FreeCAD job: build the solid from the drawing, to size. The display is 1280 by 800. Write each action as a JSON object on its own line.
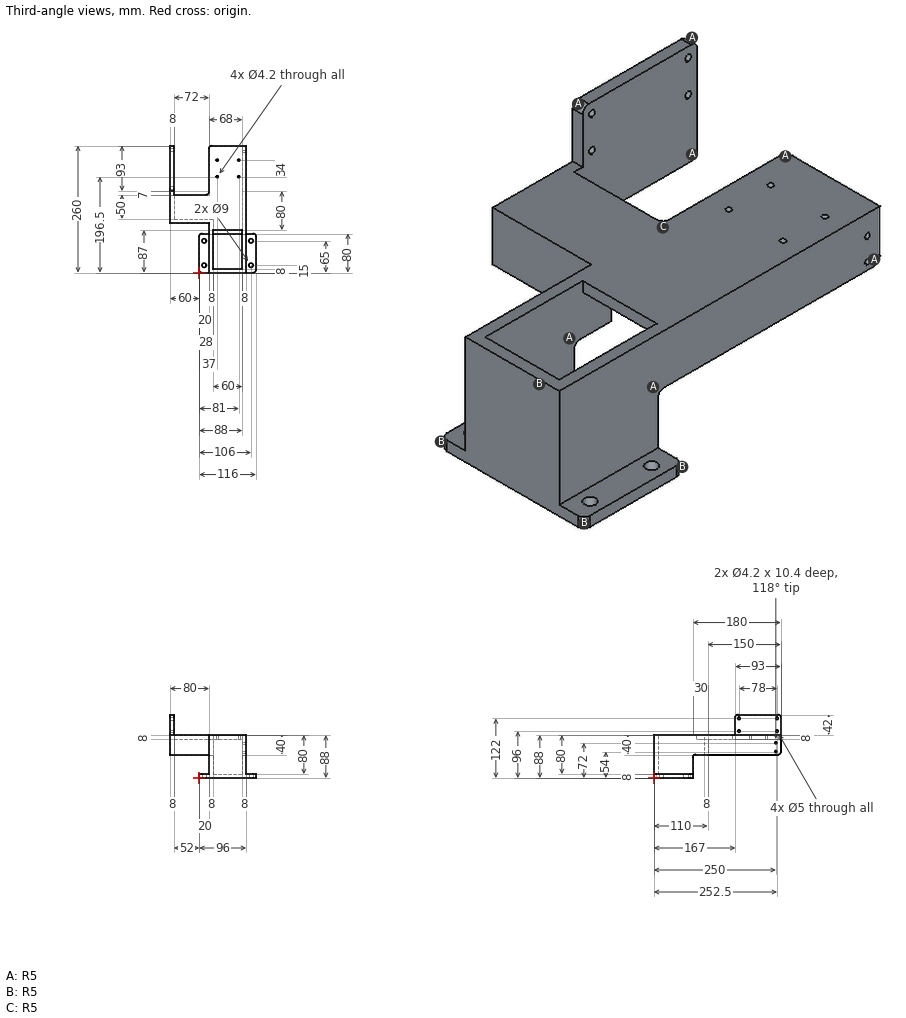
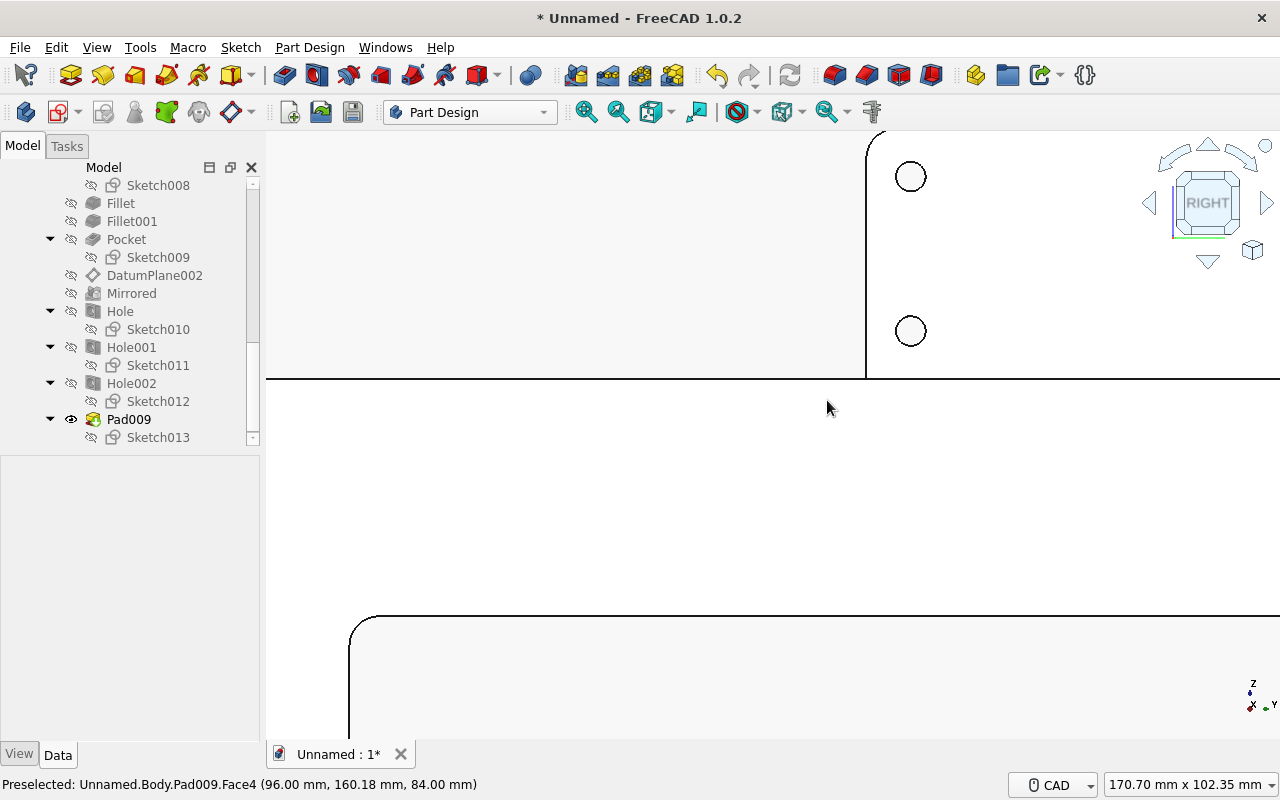
{"action": "left_click", "coordinate": [588, 112]}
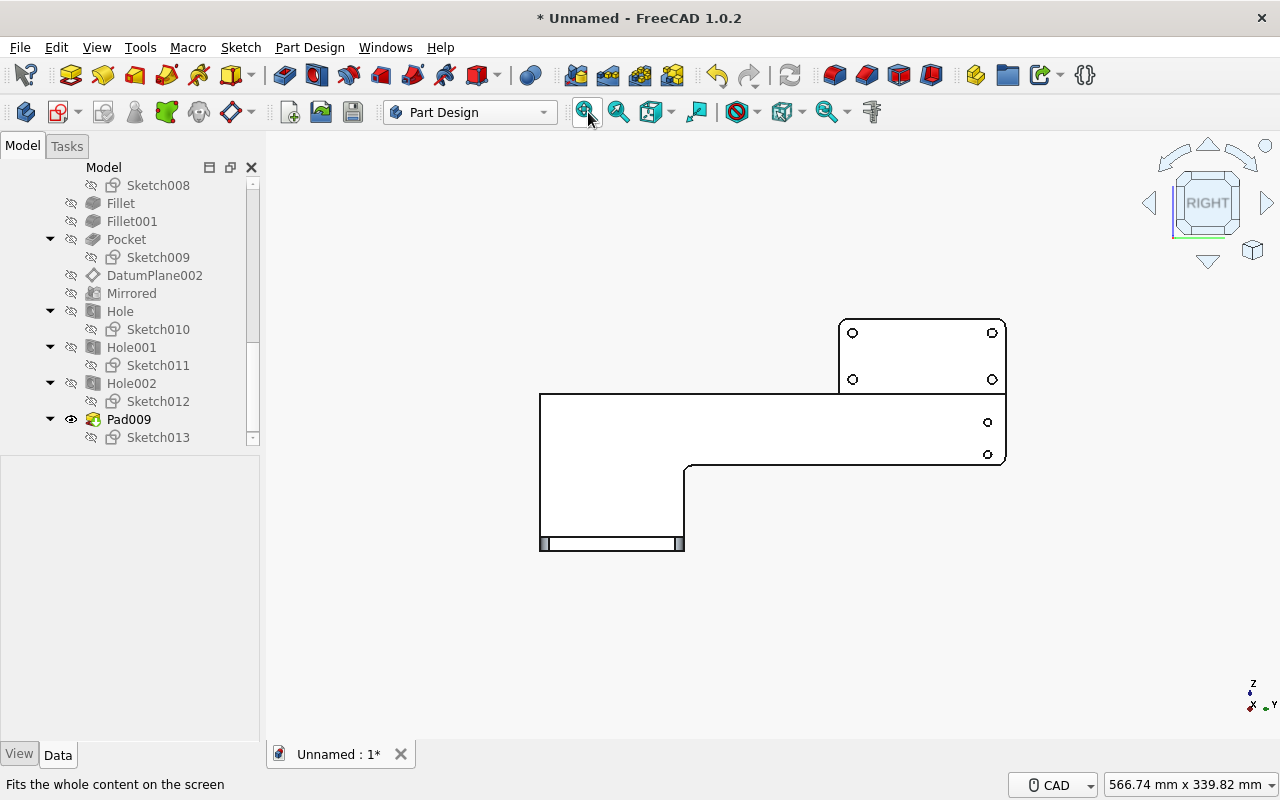
{"action": "key", "text": "5"}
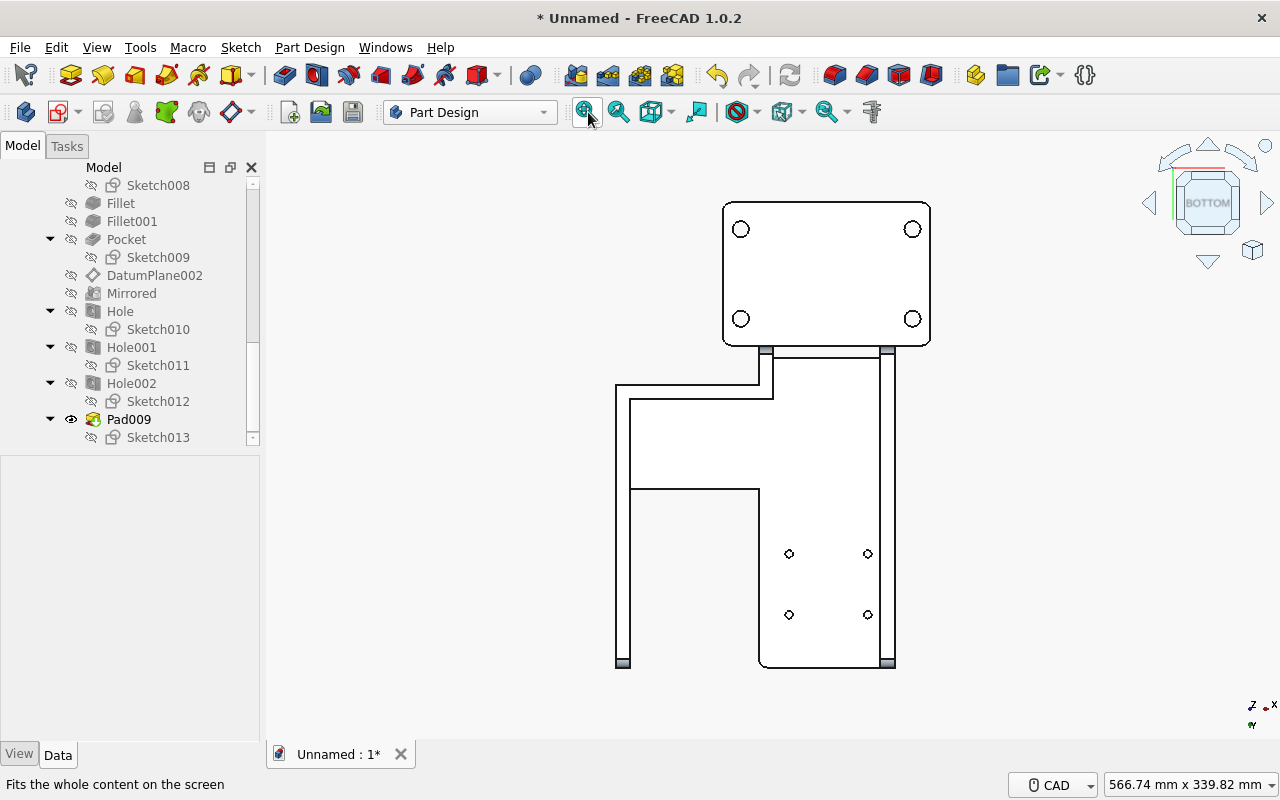
{"action": "scroll", "coordinate": [759, 488], "scroll_direction": "up", "scroll_amount": 6}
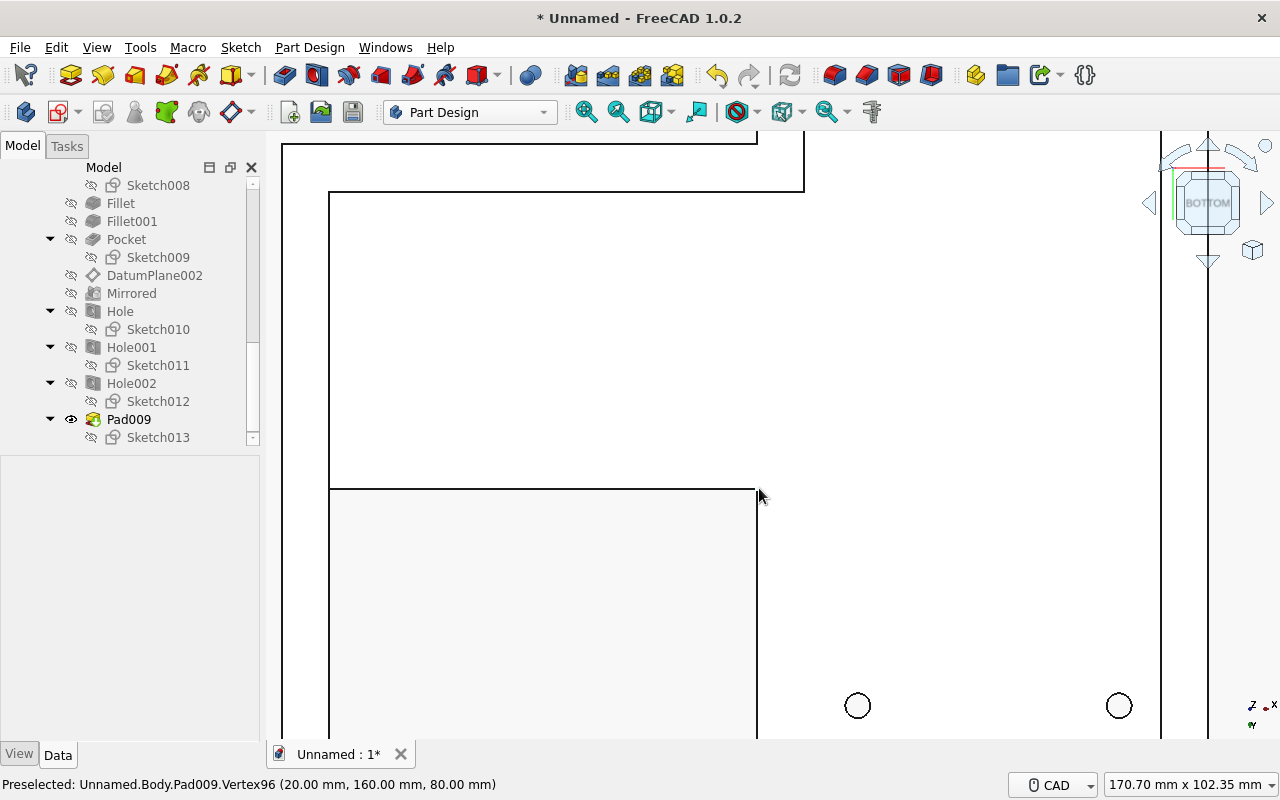
{"action": "left_click", "coordinate": [588, 112]}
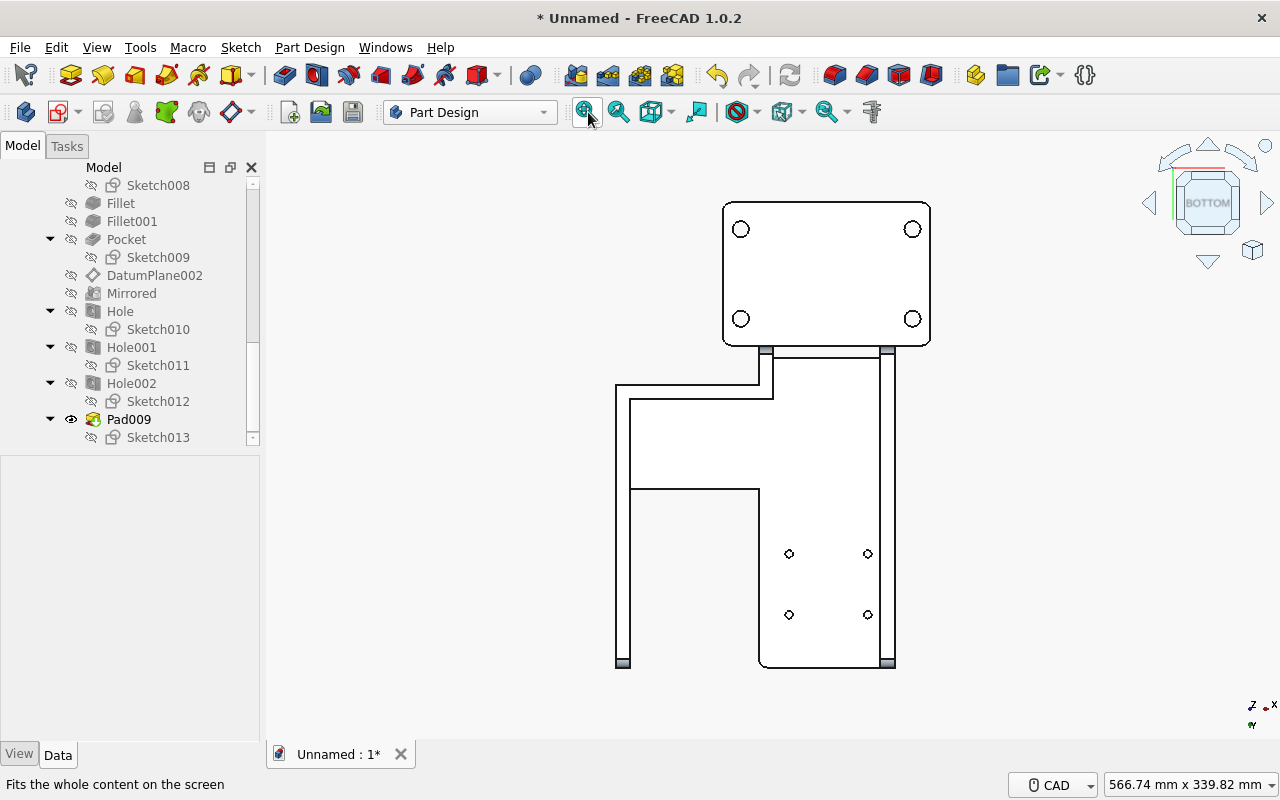
{"action": "key", "text": "4"}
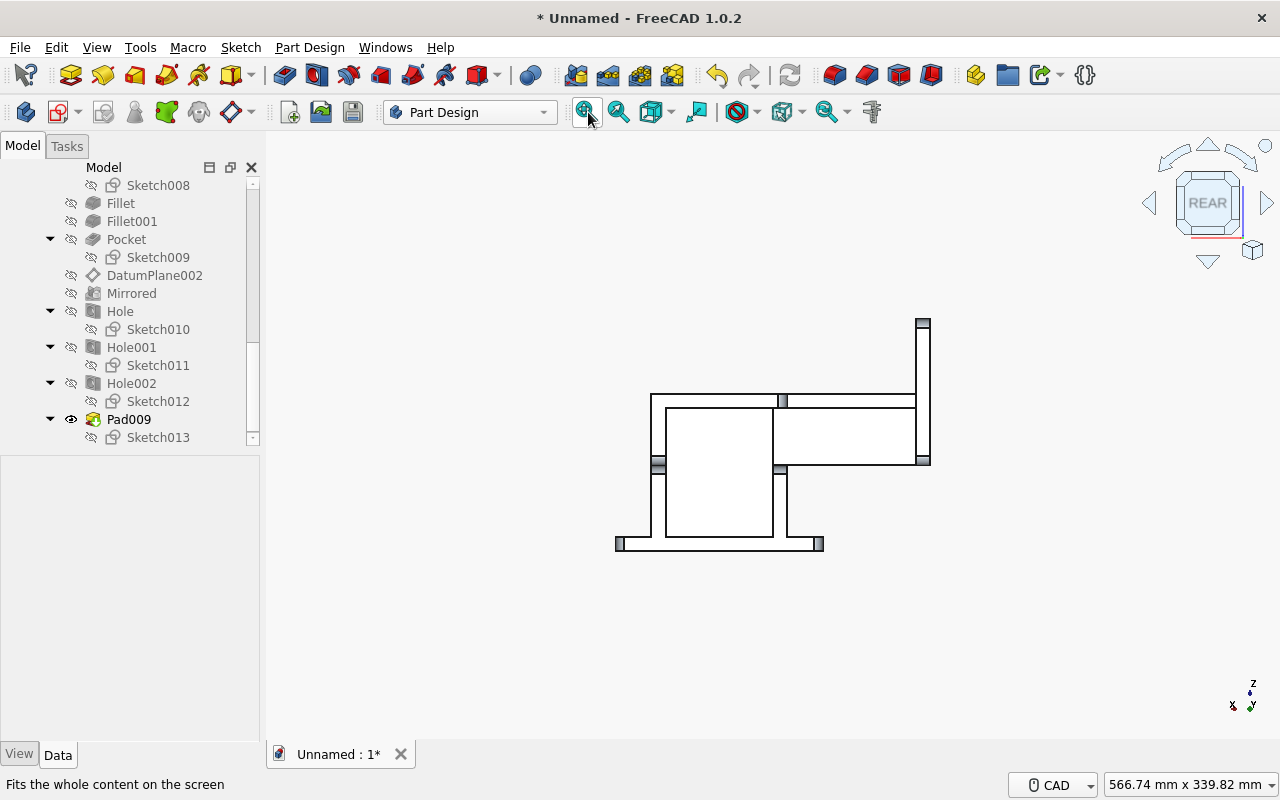
{"action": "left_click", "coordinate": [588, 112]}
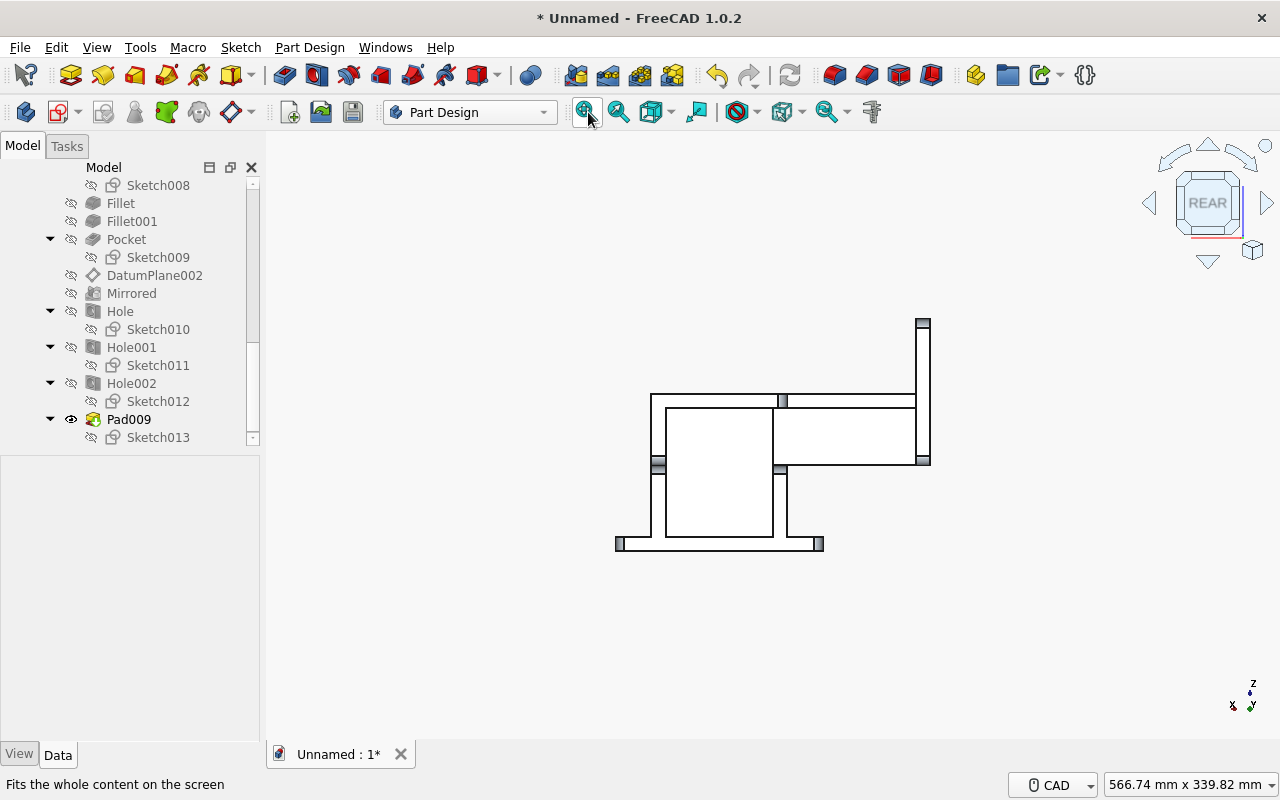
{"action": "scroll", "coordinate": [787, 400], "scroll_direction": "up", "scroll_amount": 6}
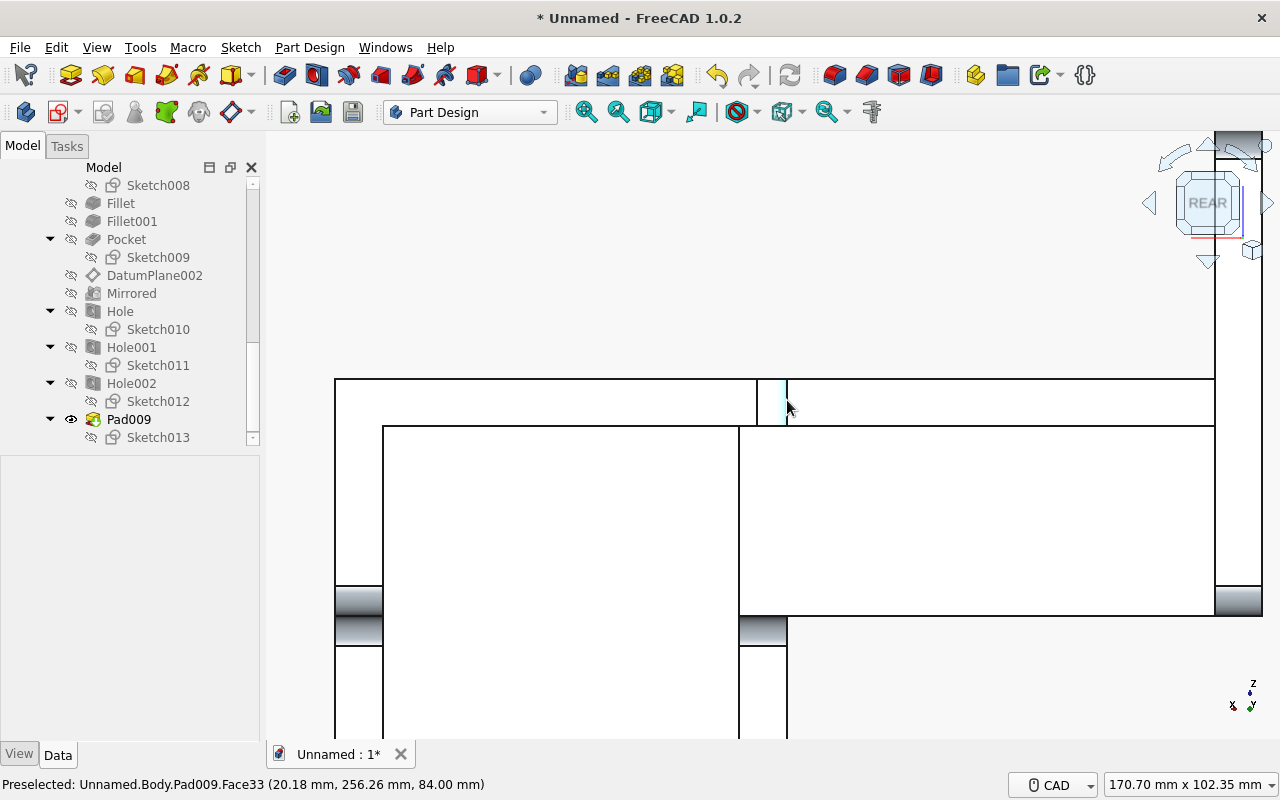
{"action": "left_click", "coordinate": [588, 112]}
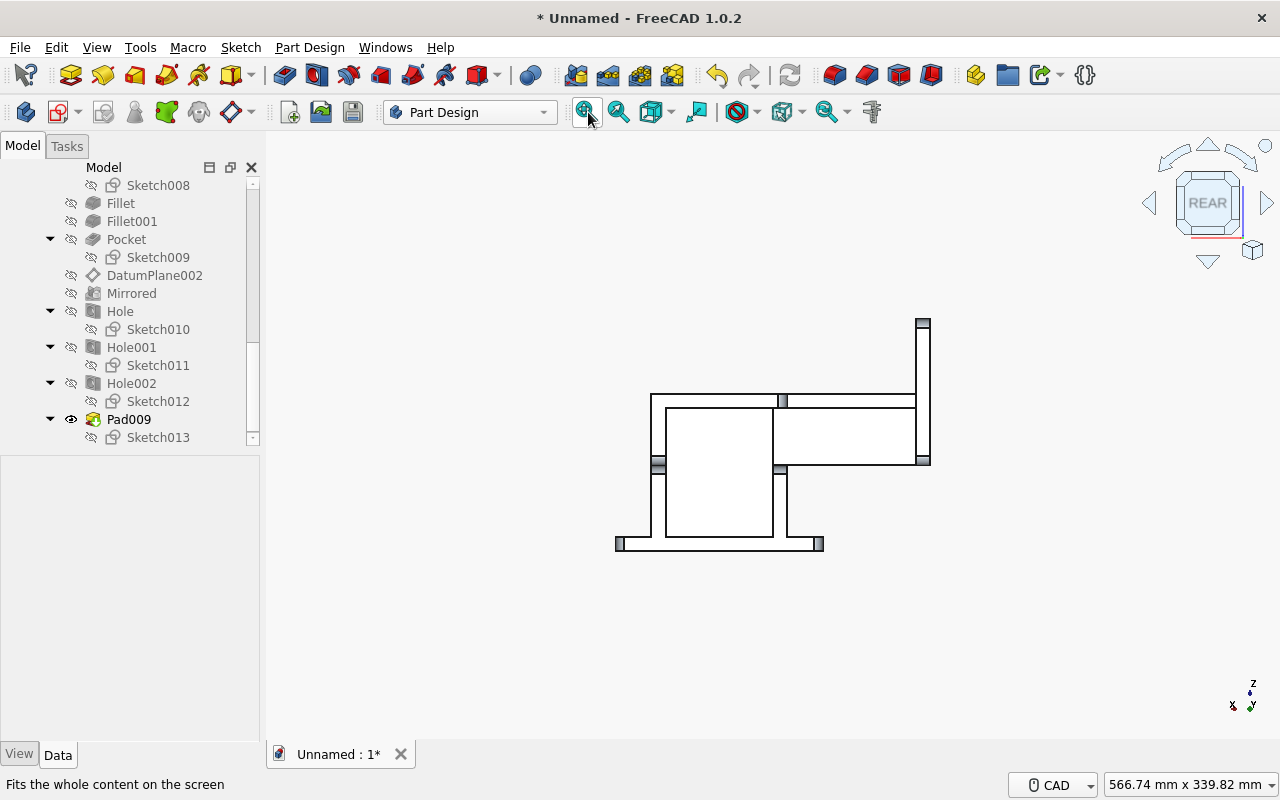
{"action": "key", "text": "6"}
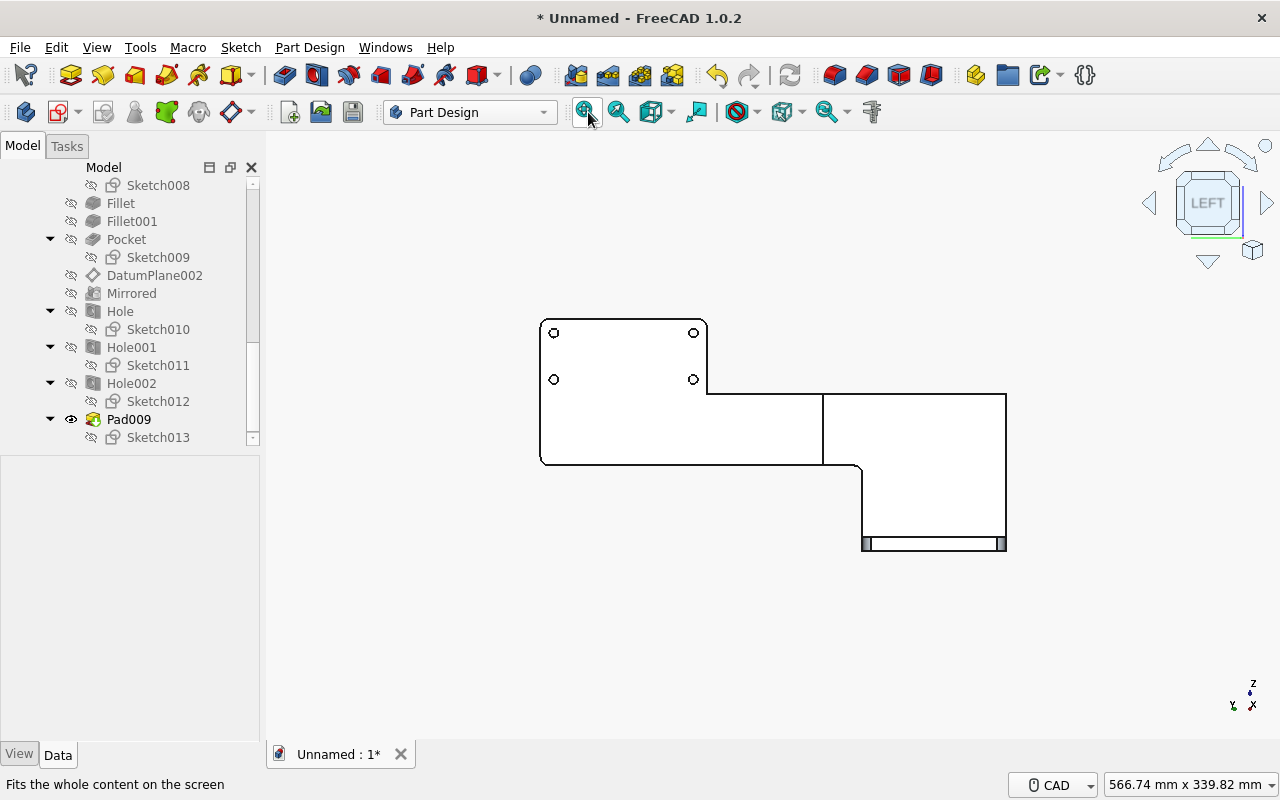
{"action": "scroll", "coordinate": [719, 400], "scroll_direction": "up", "scroll_amount": 6}